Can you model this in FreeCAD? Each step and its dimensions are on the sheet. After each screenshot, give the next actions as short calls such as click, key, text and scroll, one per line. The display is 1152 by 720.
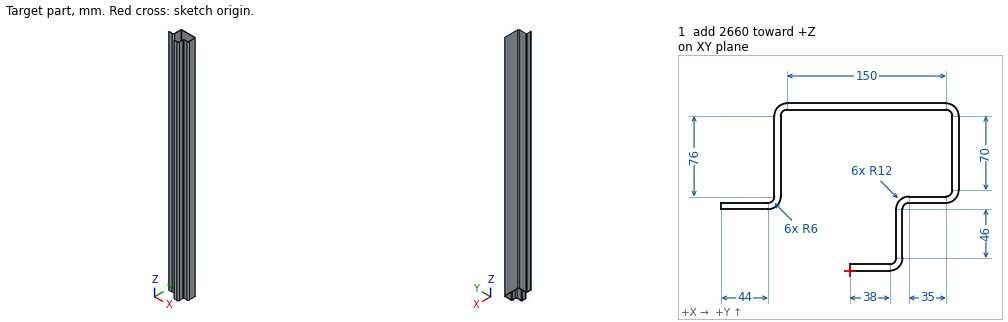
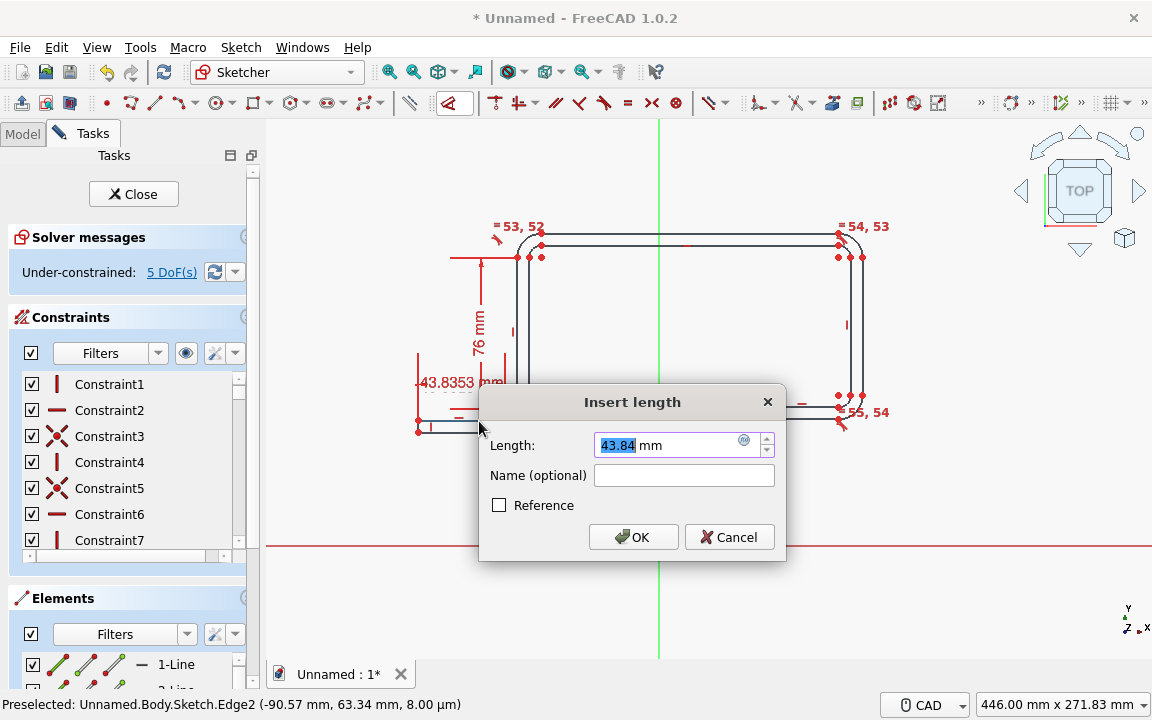
text(44)
key(Return)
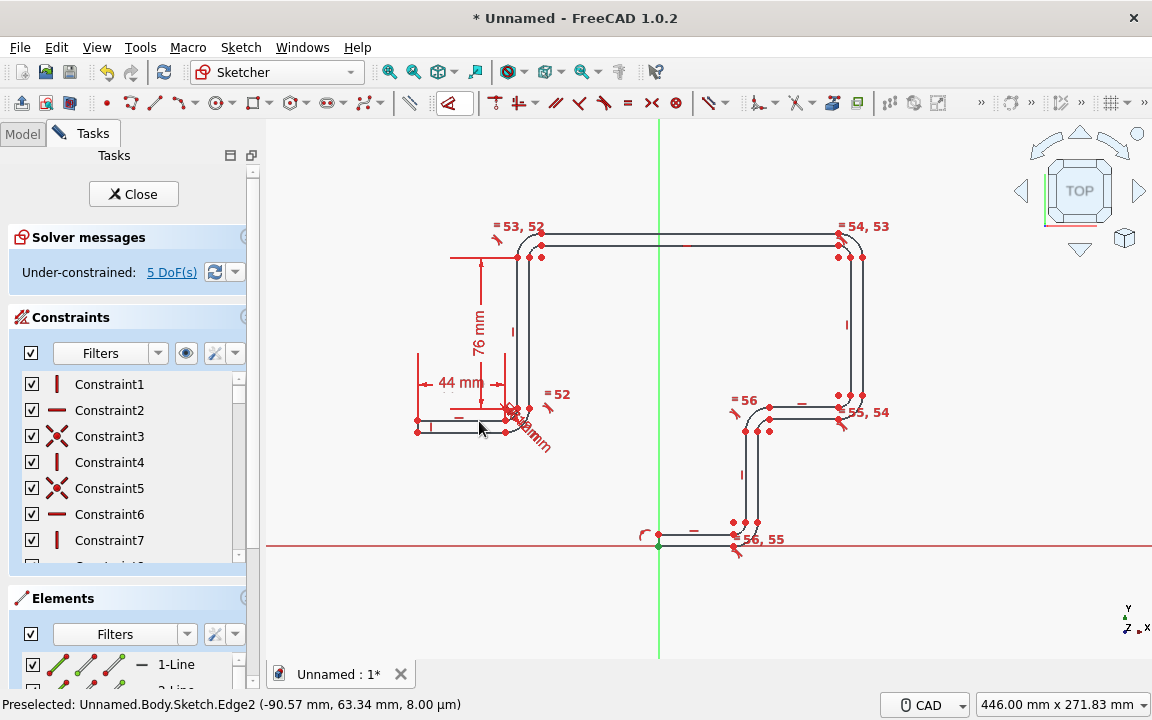
click(851, 299)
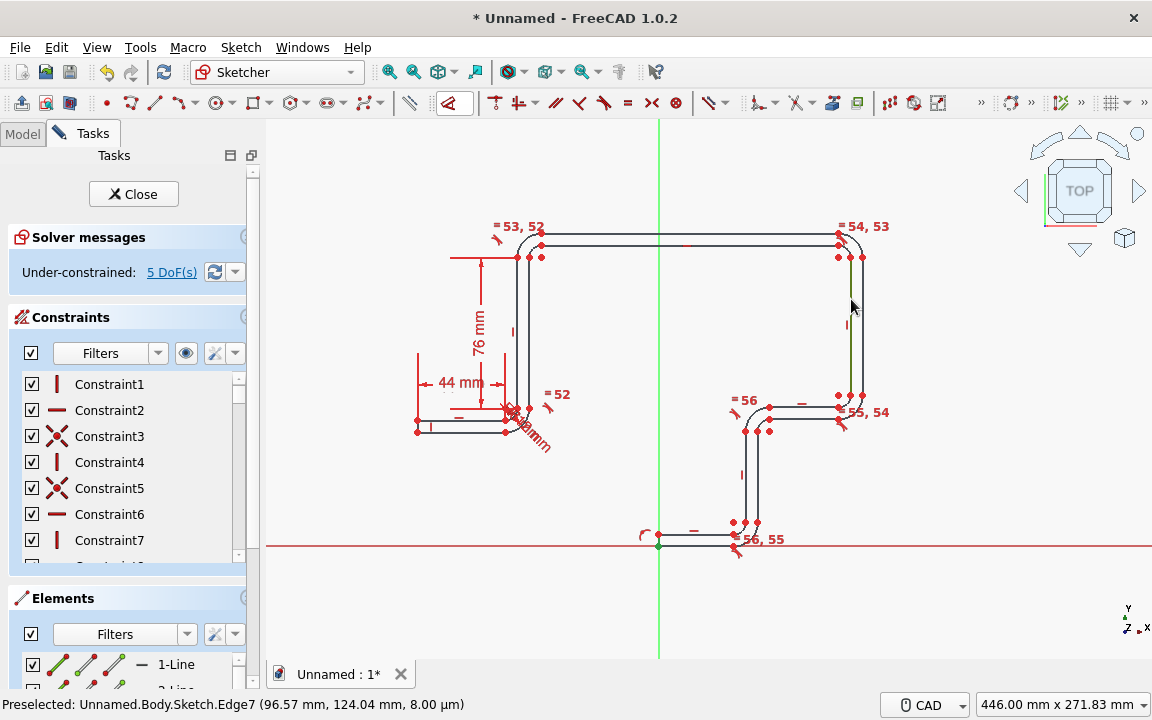
key(i)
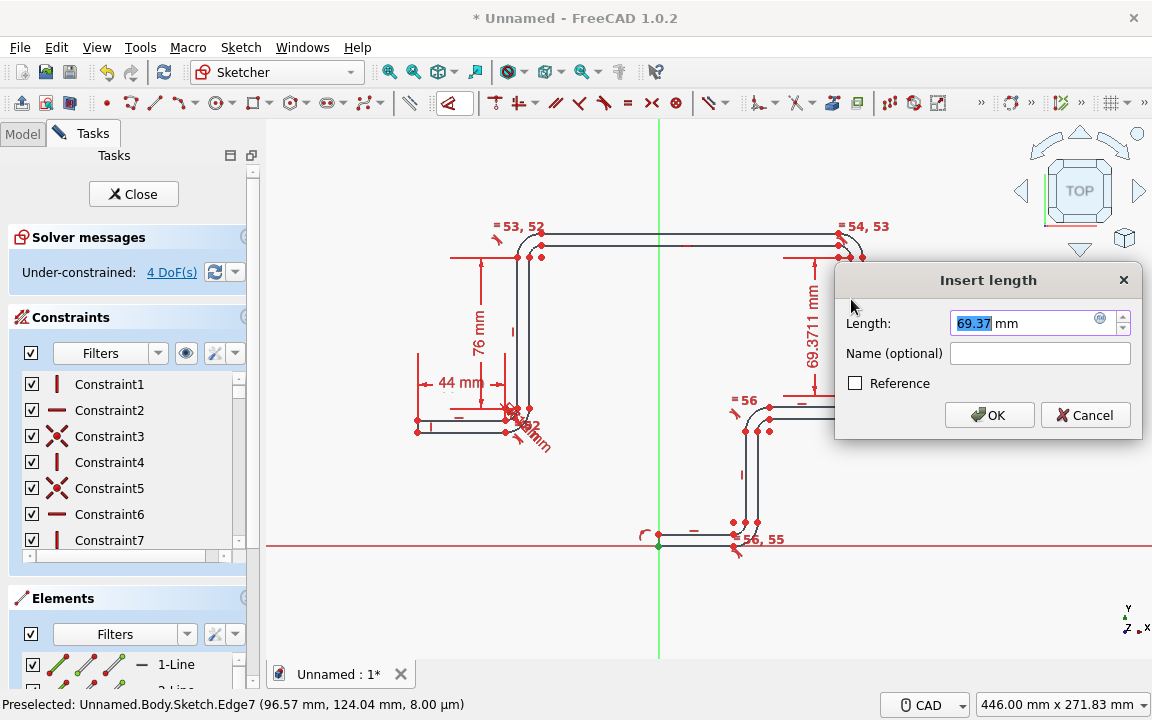
text(70)
key(Return)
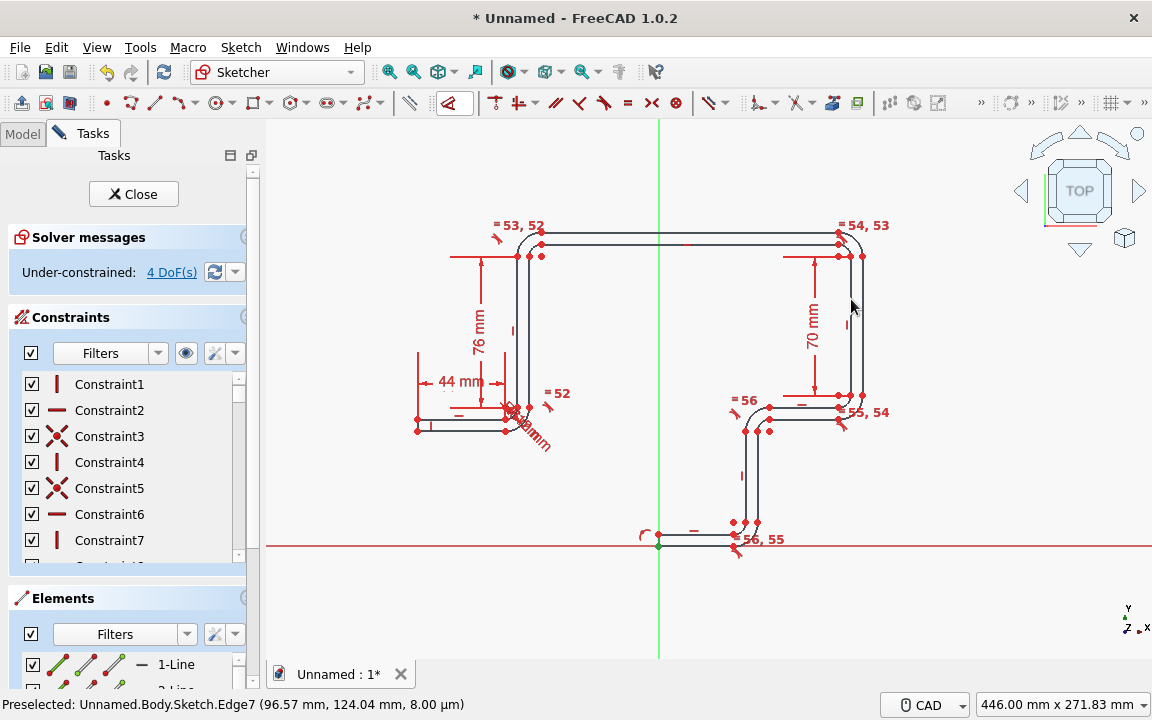
click(818, 408)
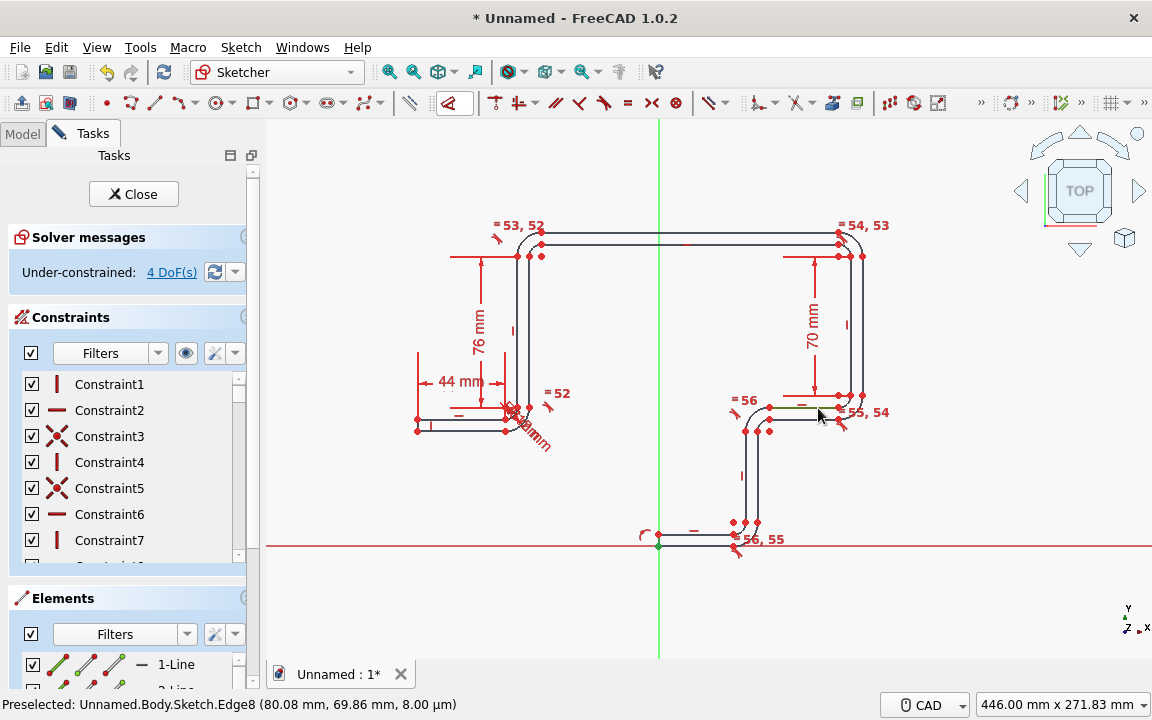
key(l)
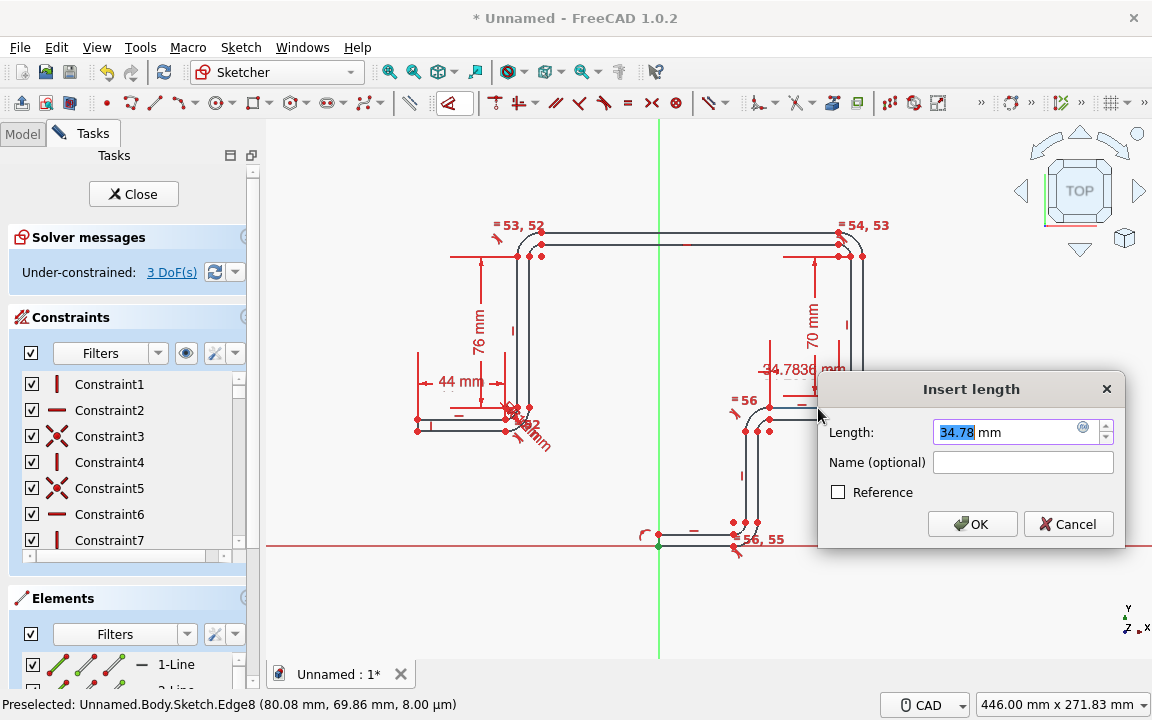
text(35)
key(Return)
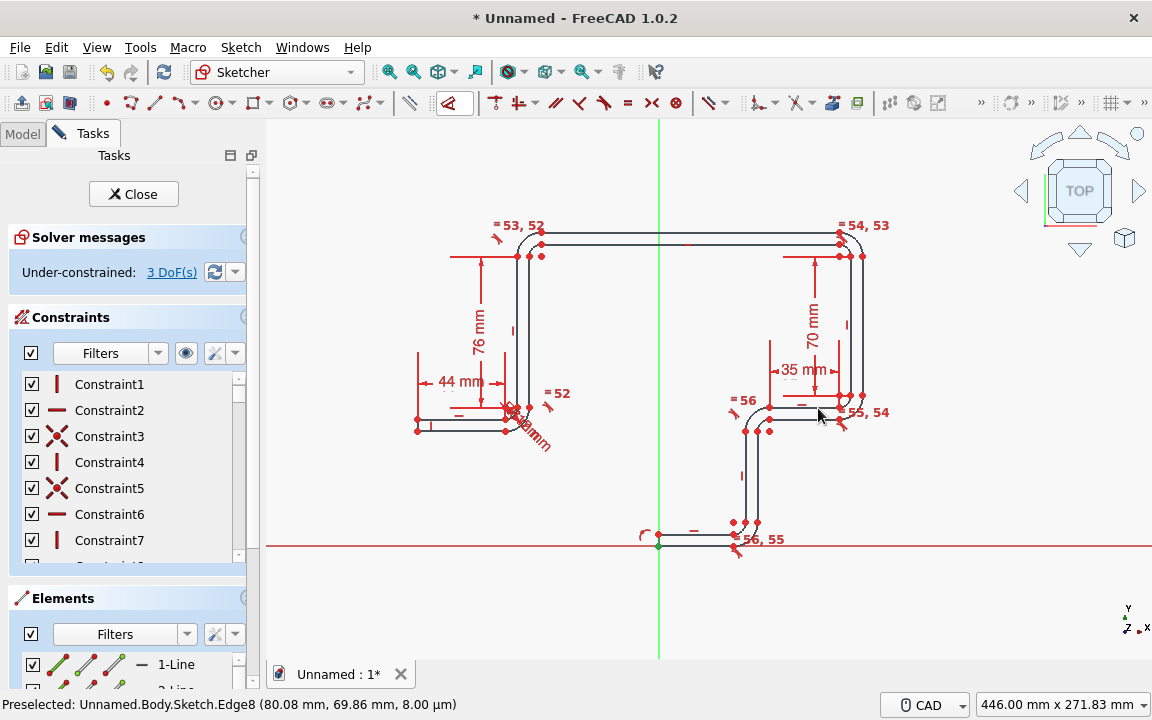
click(746, 459)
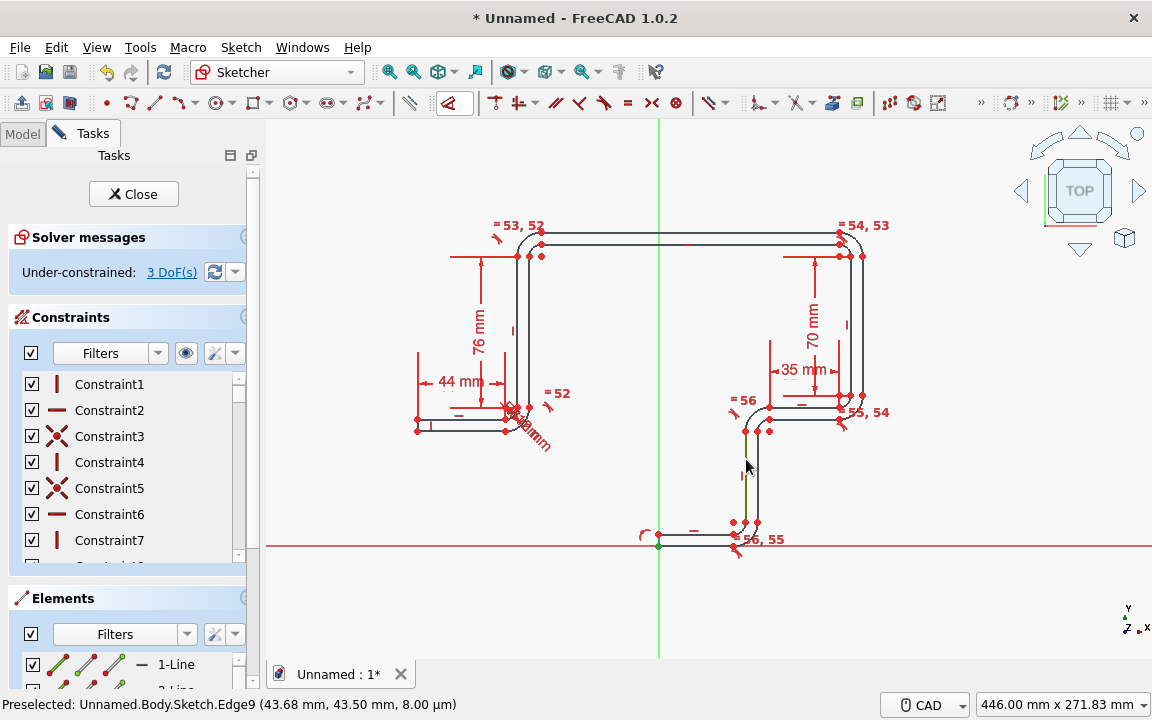
key(i)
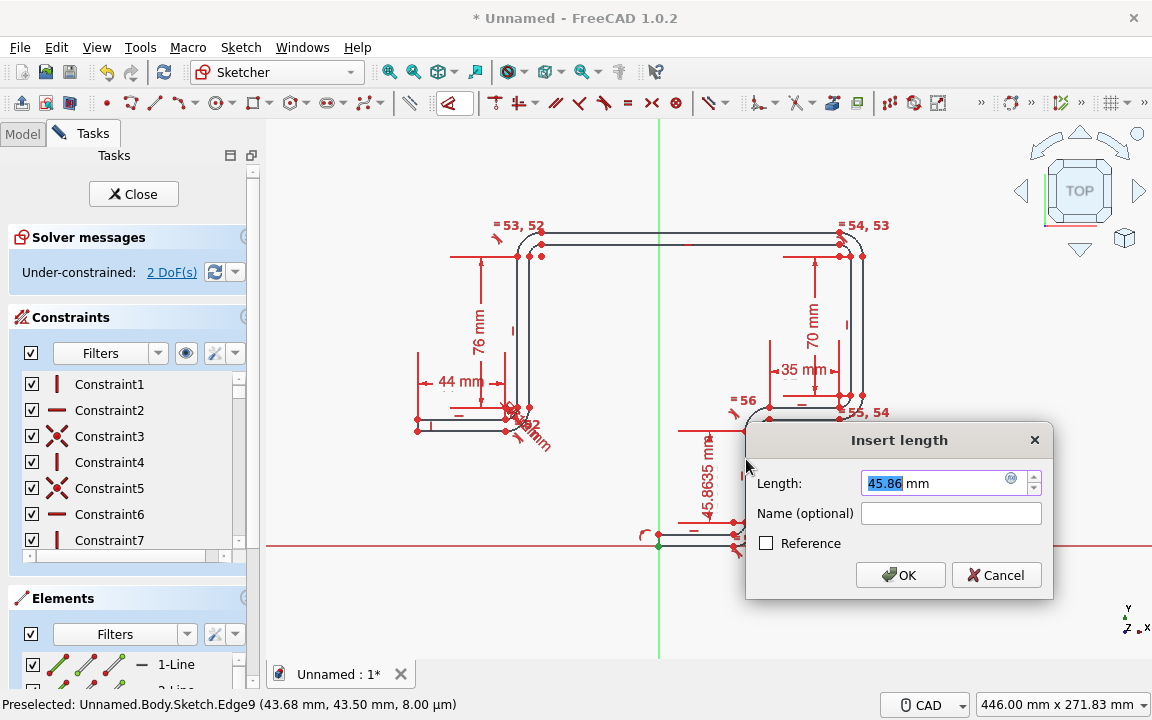
text(46)
key(Return)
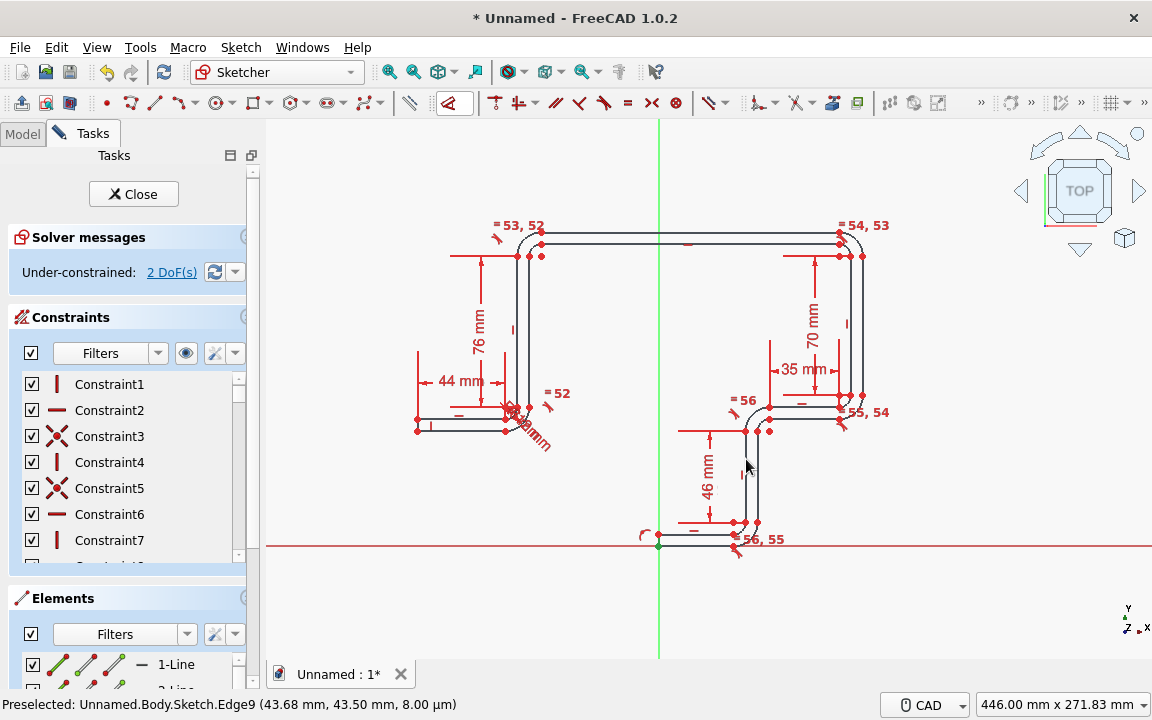
click(711, 534)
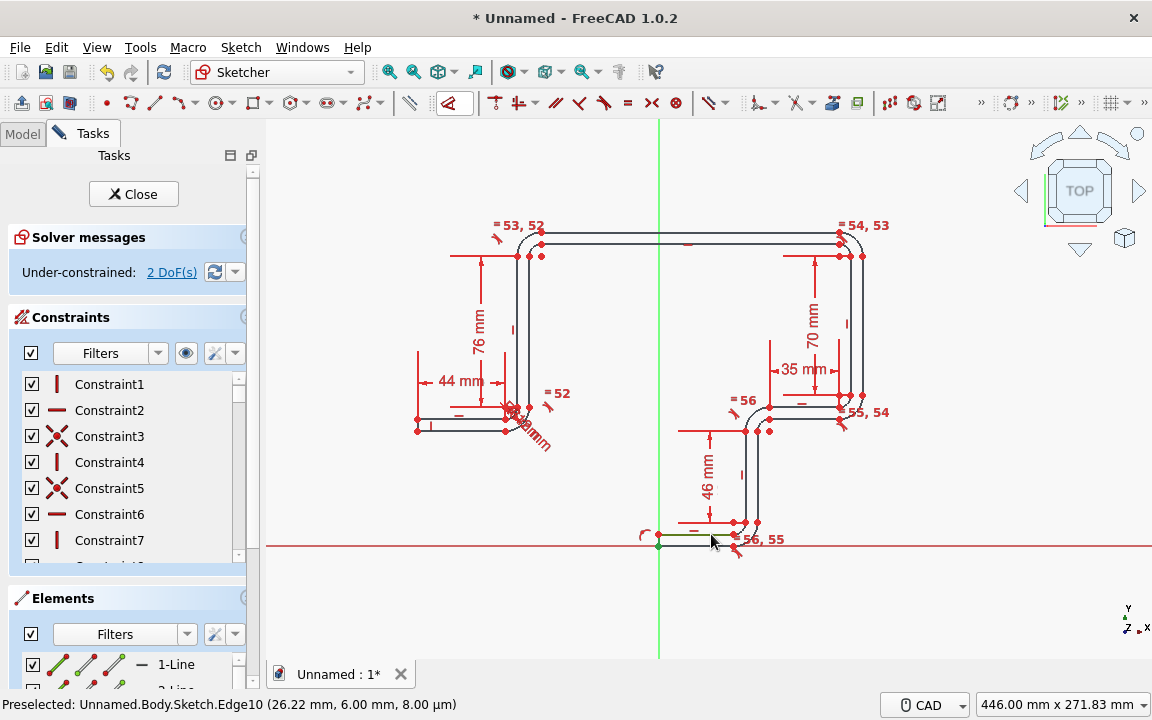
click(468, 104)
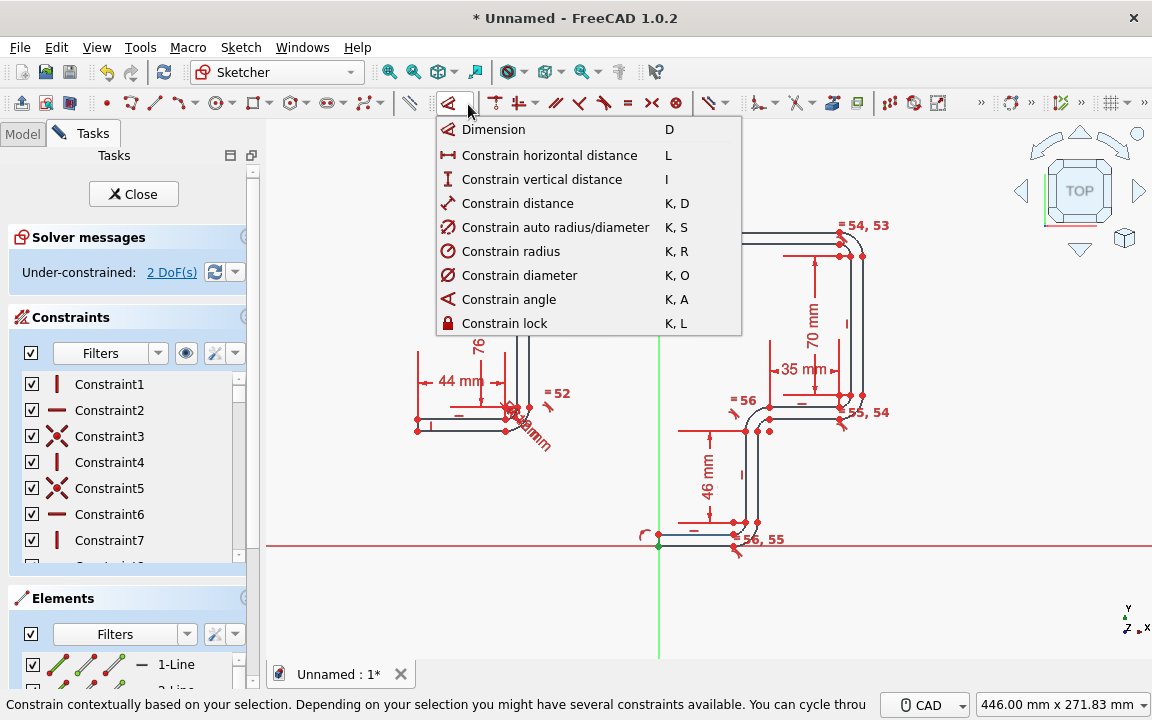
click(589, 155)